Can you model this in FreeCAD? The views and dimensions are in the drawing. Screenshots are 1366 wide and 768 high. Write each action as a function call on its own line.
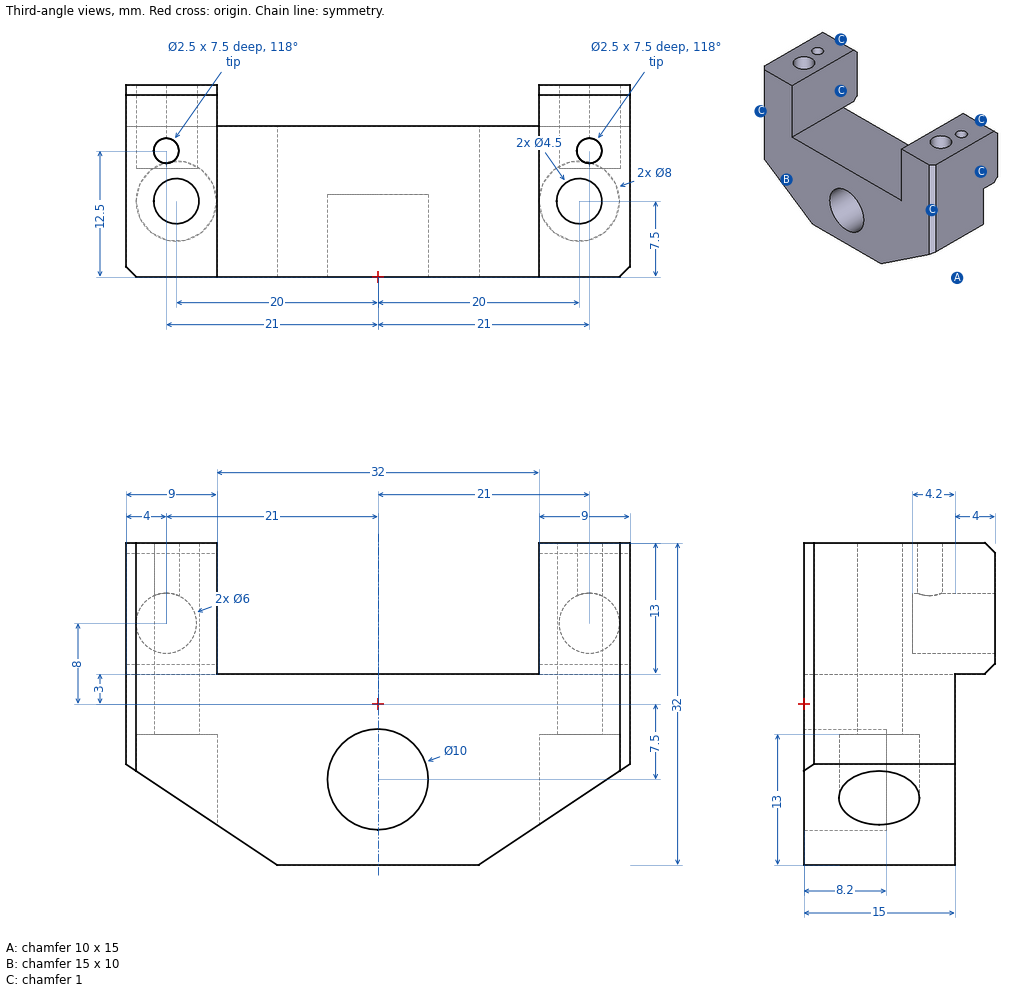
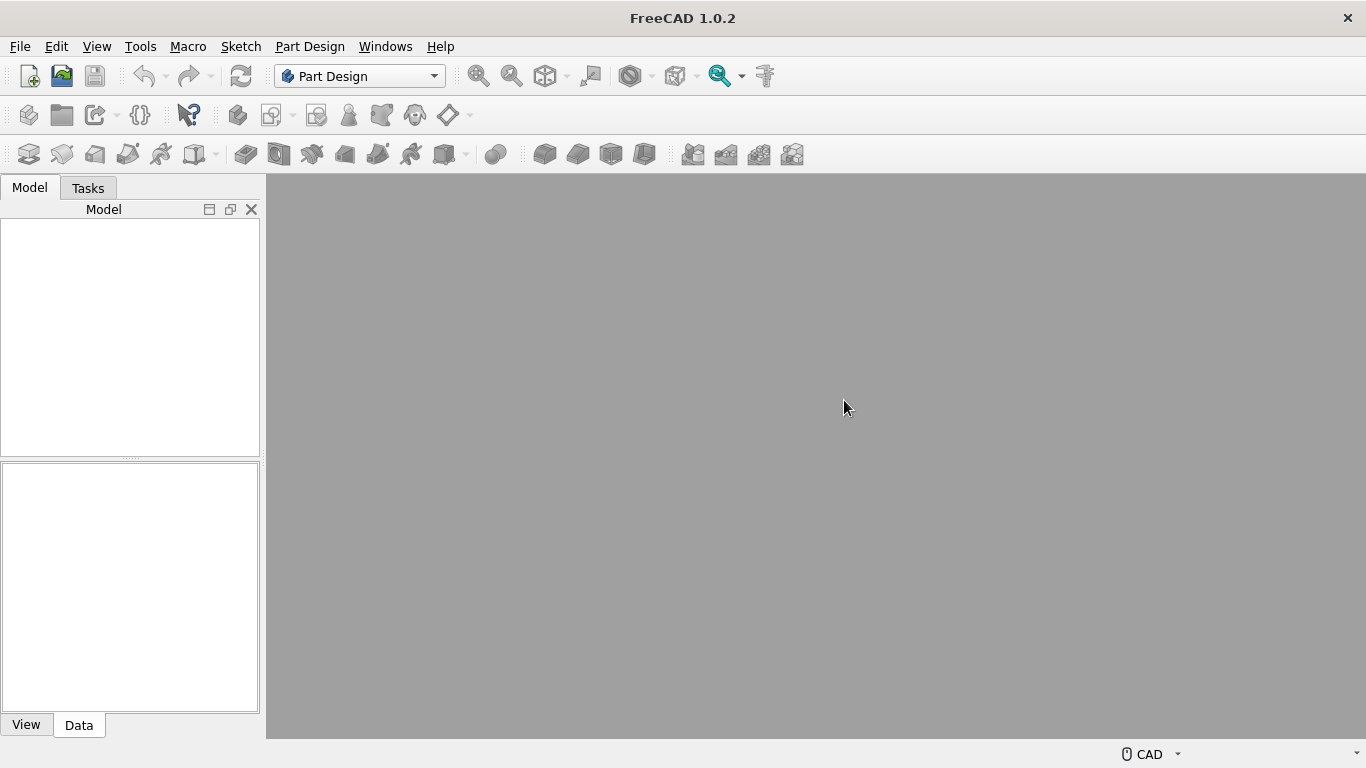
click(29, 76)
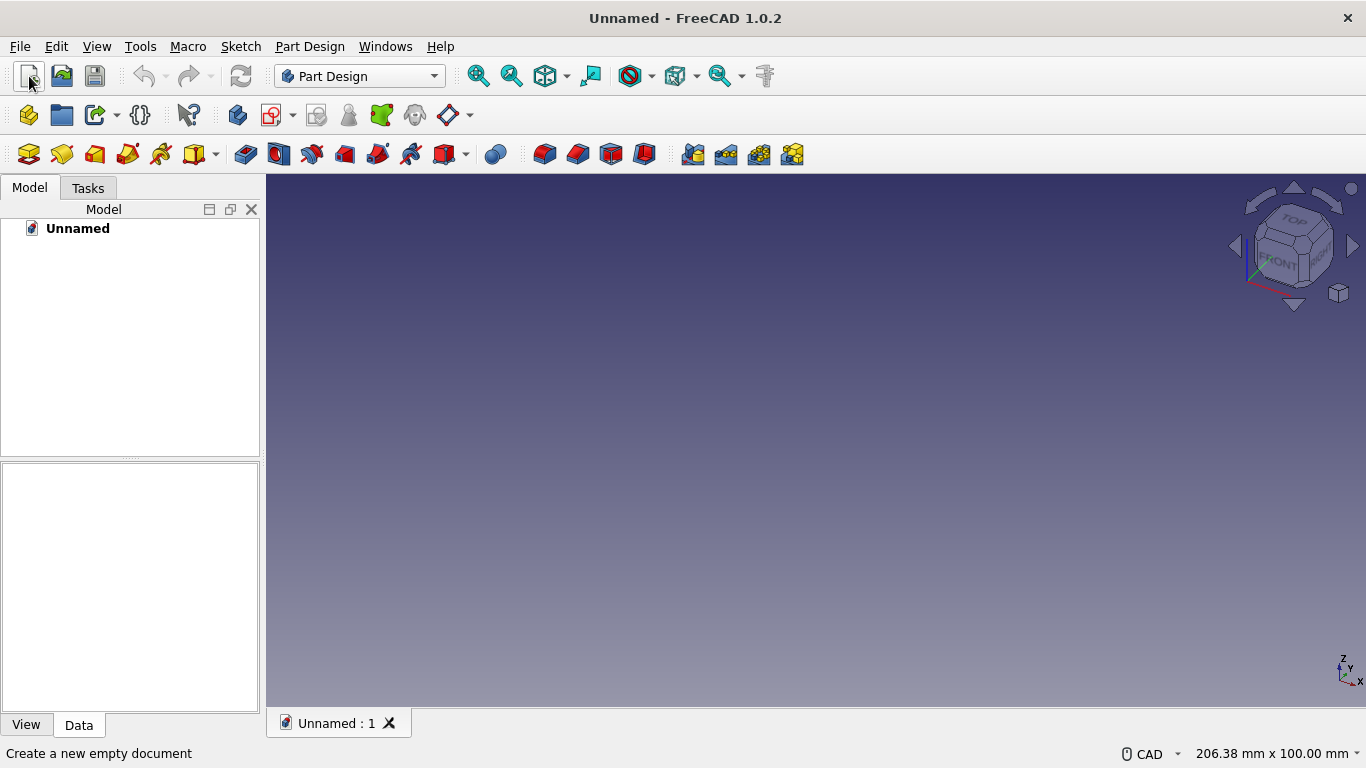
click(270, 116)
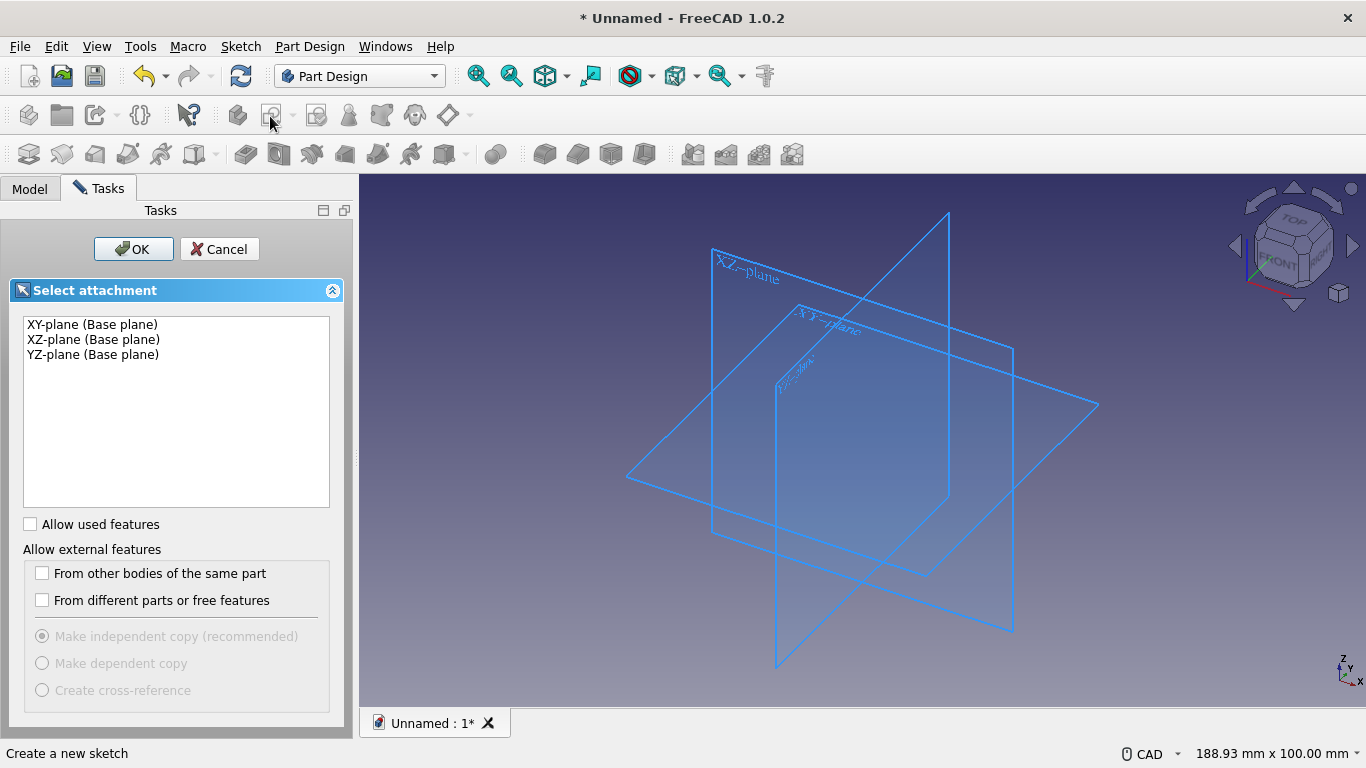
click(84, 340)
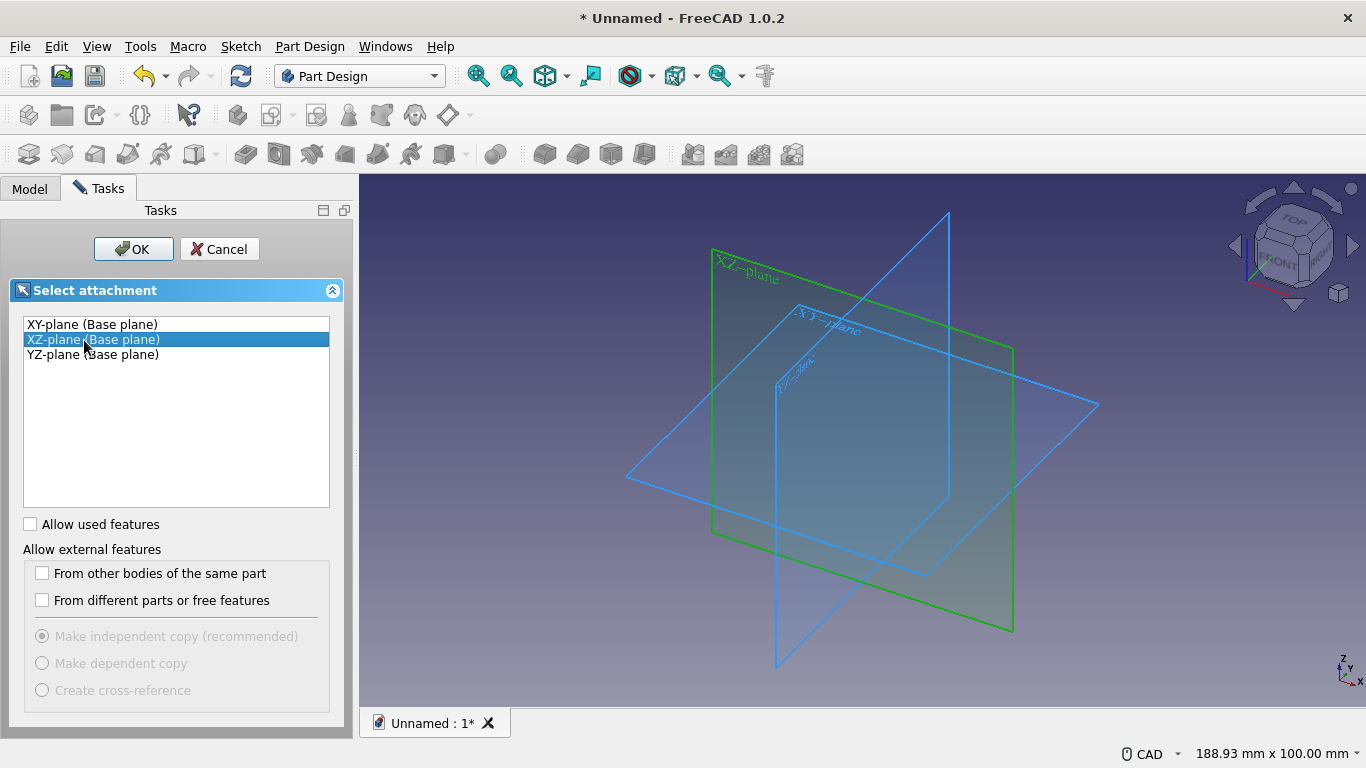
click(134, 249)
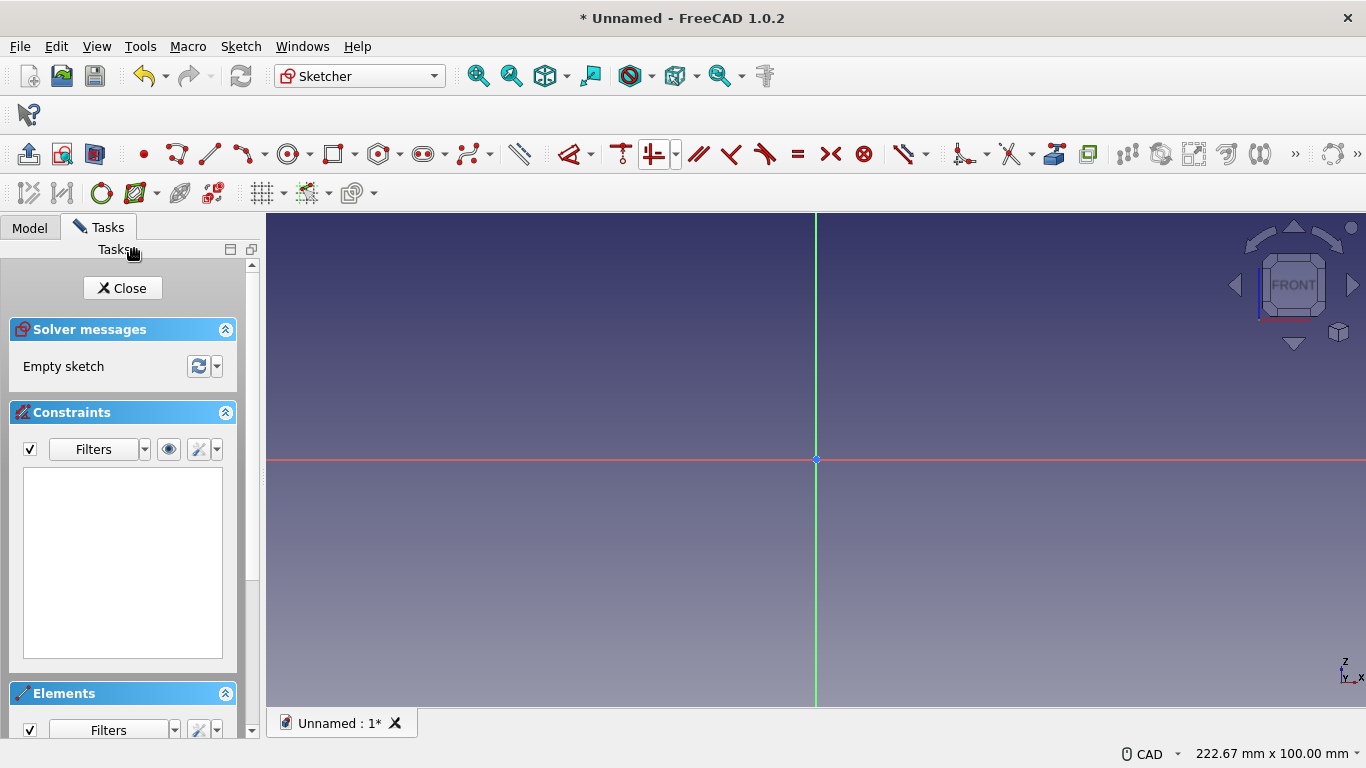
scroll(899, 460, up, 3)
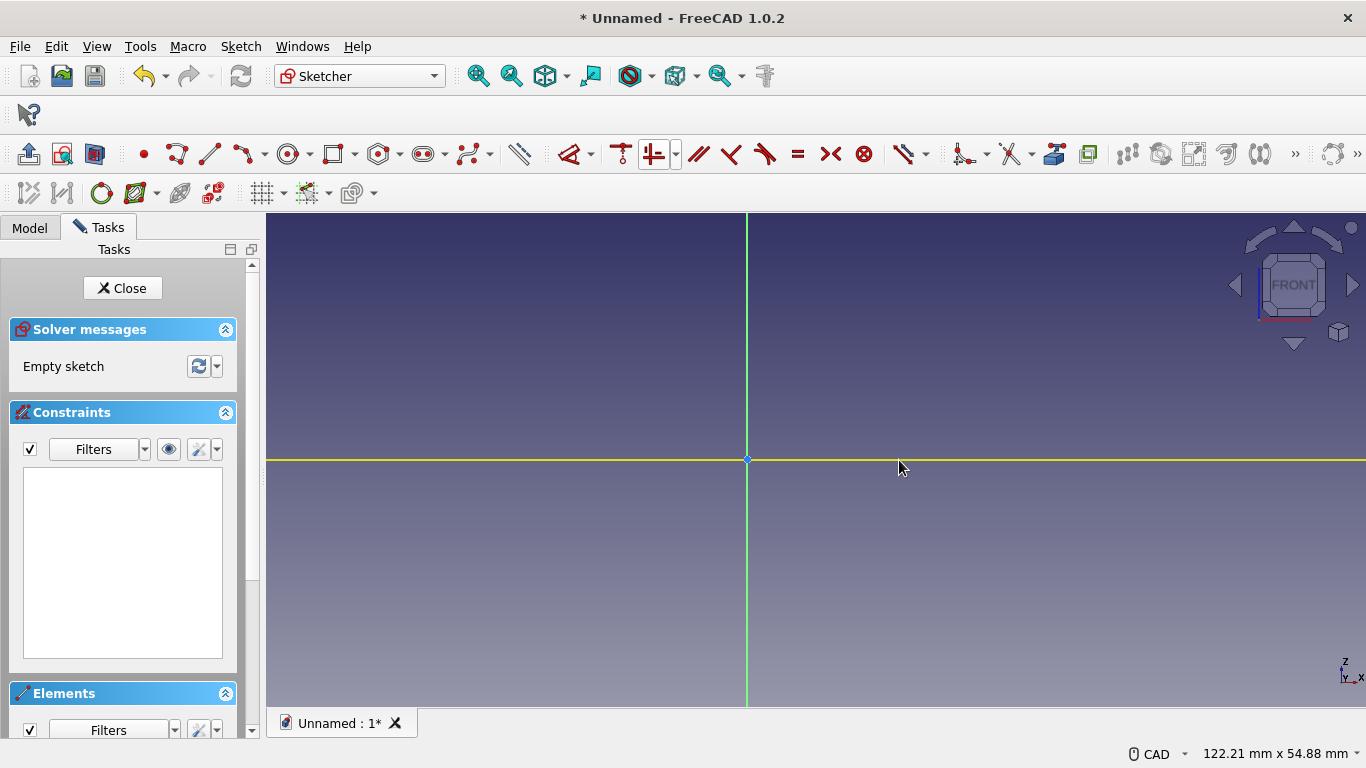
click(177, 154)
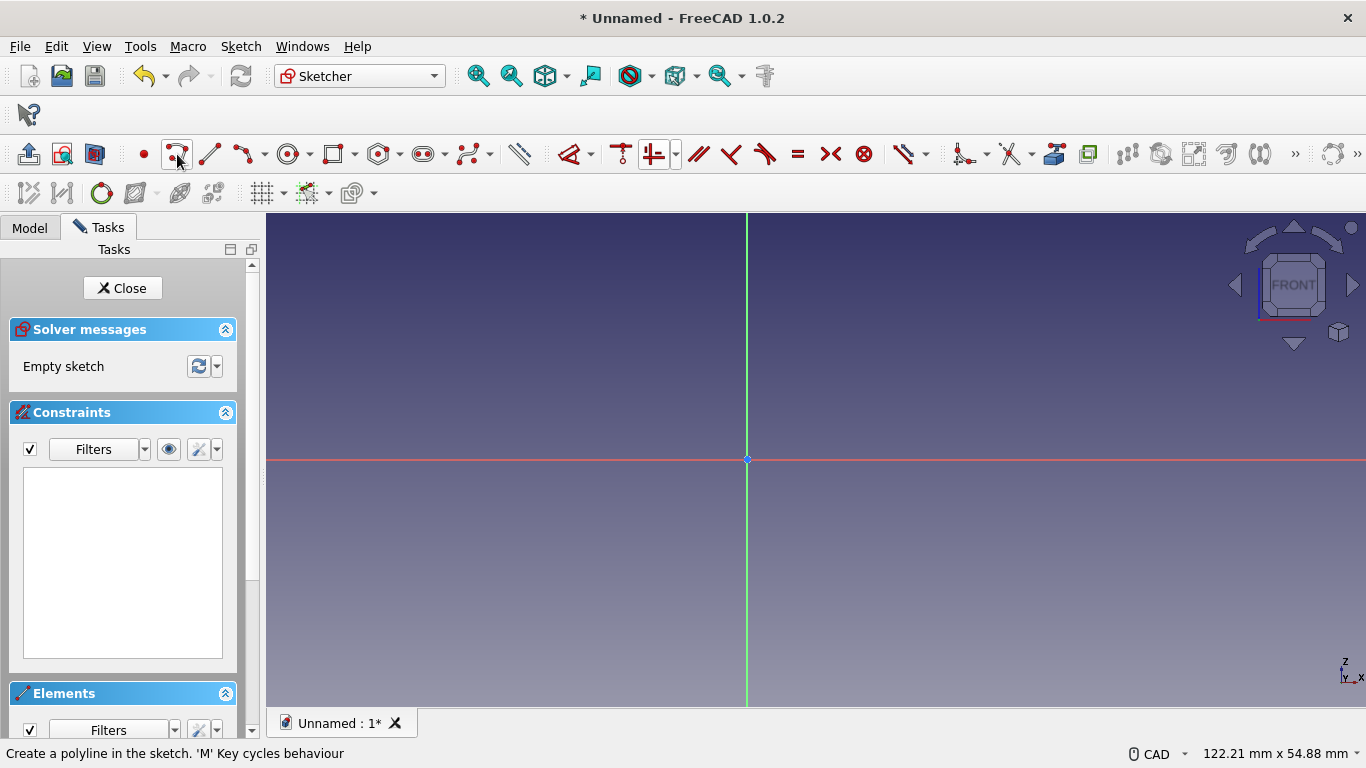
click(603, 433)
click(891, 433)
click(891, 316)
click(972, 316)
click(972, 604)
click(522, 604)
click(522, 316)
click(603, 316)
click(603, 434)
key(Escape)
key(Escape)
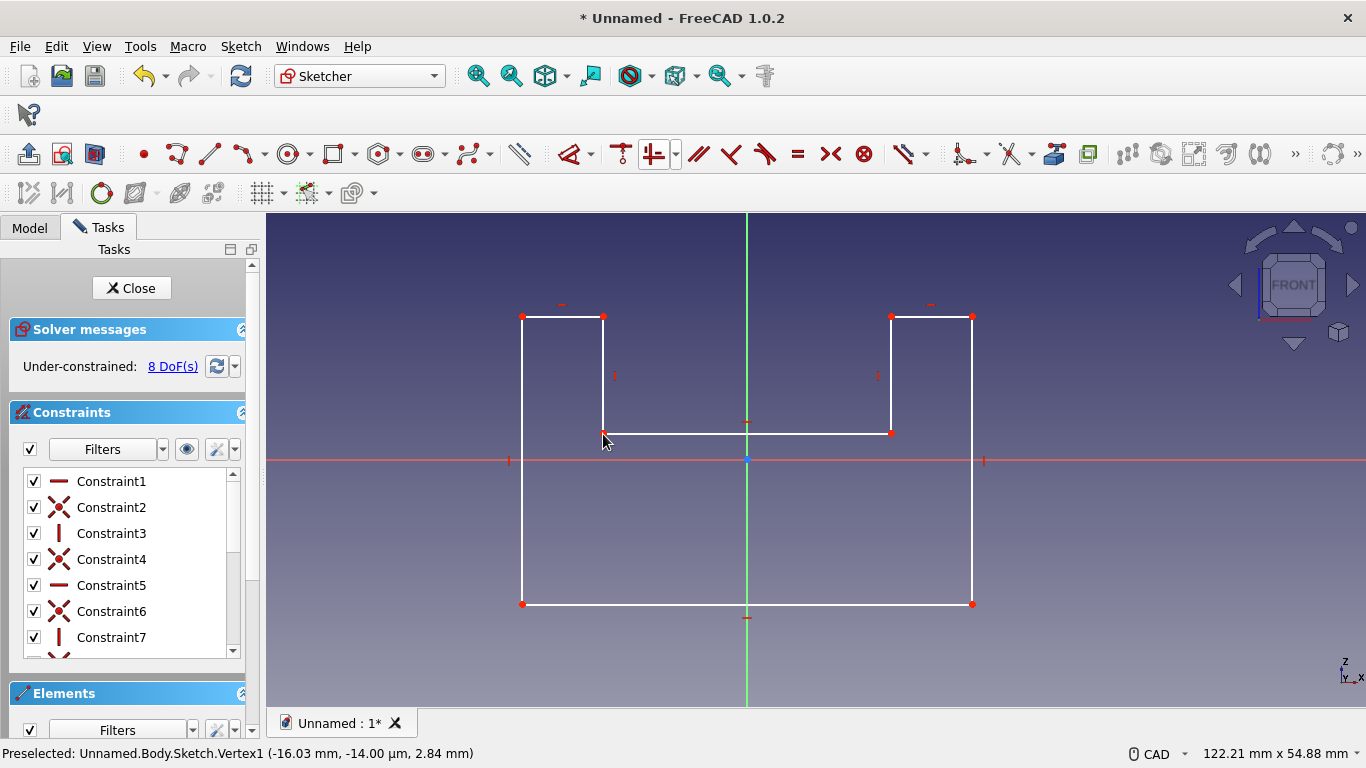
click(972, 317)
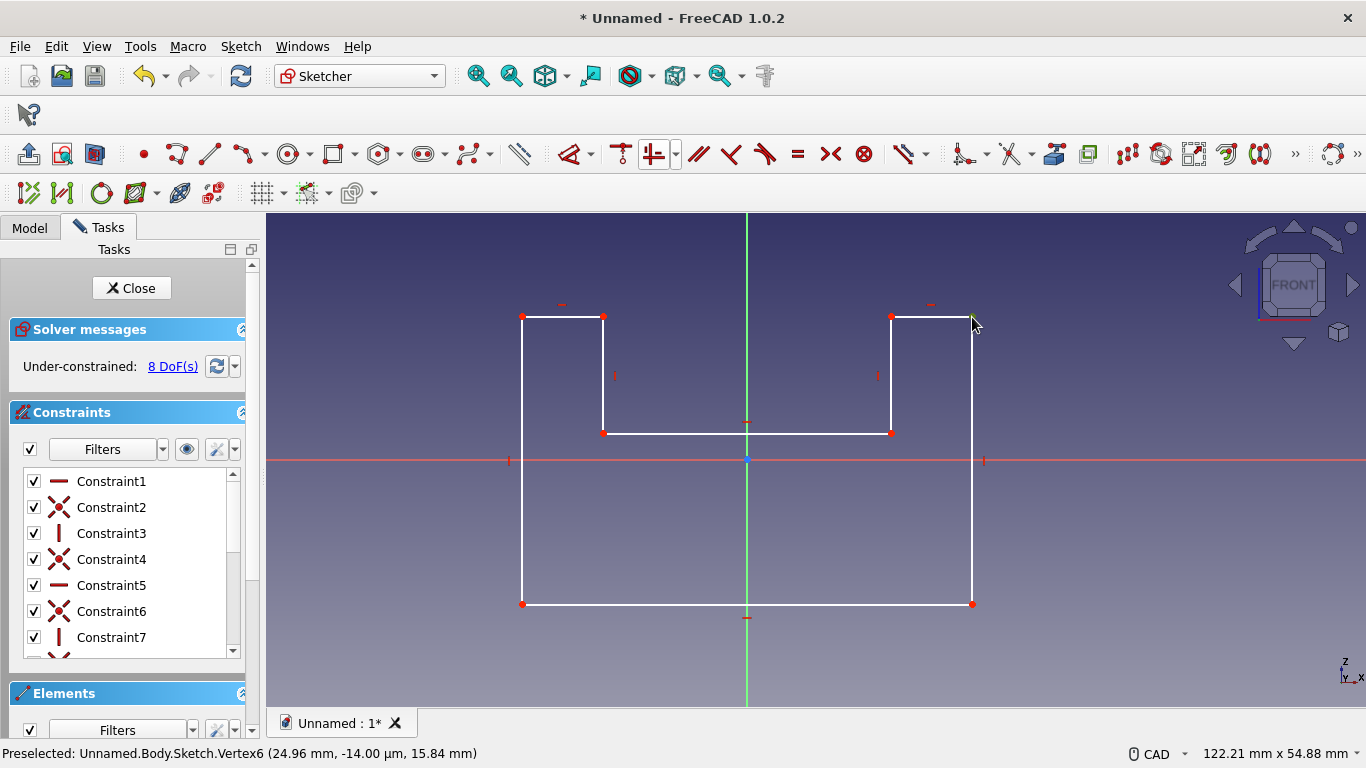
click(522, 317)